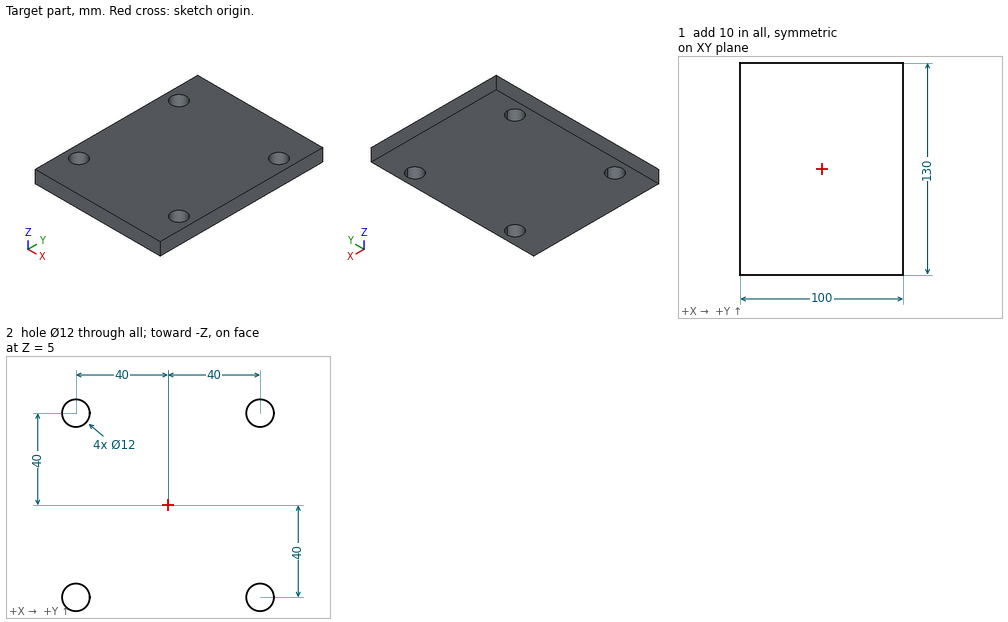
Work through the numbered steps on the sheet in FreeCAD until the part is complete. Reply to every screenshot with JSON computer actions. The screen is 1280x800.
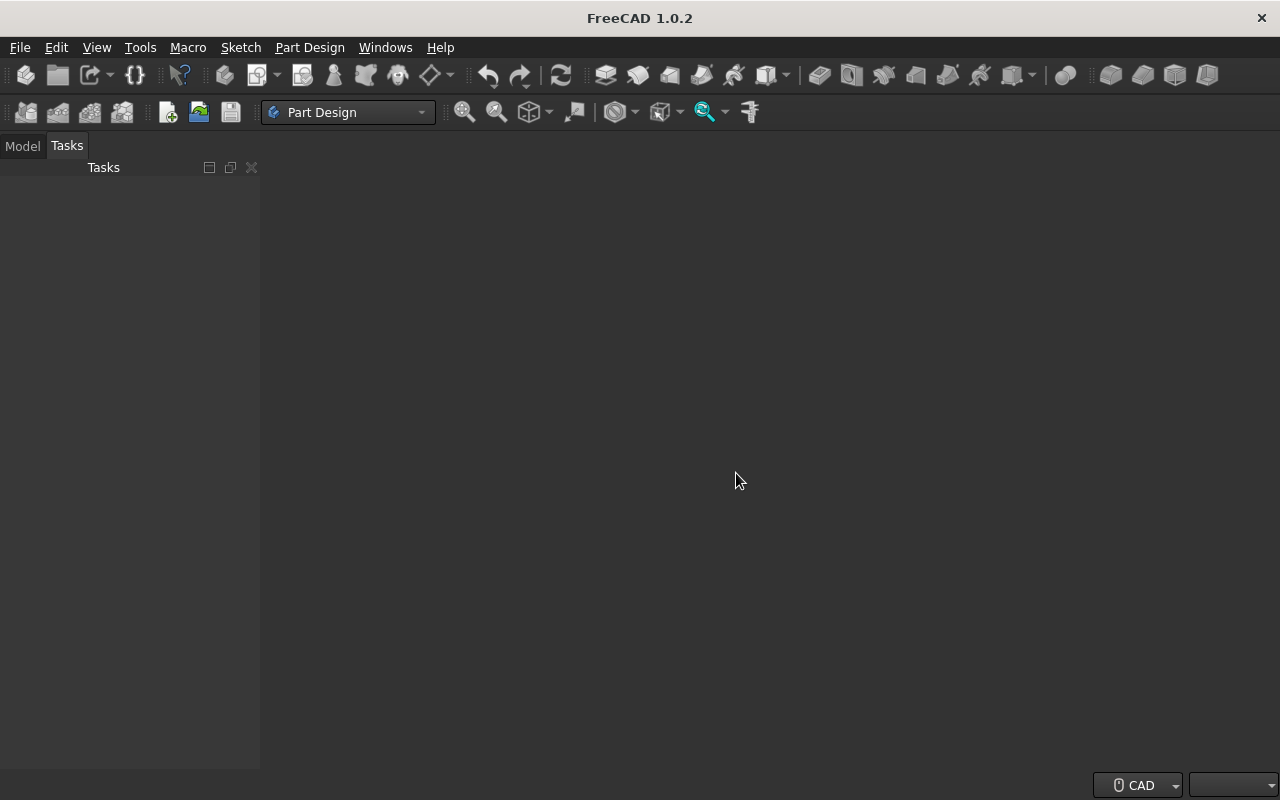
{"action": "left_click", "coordinate": [168, 112]}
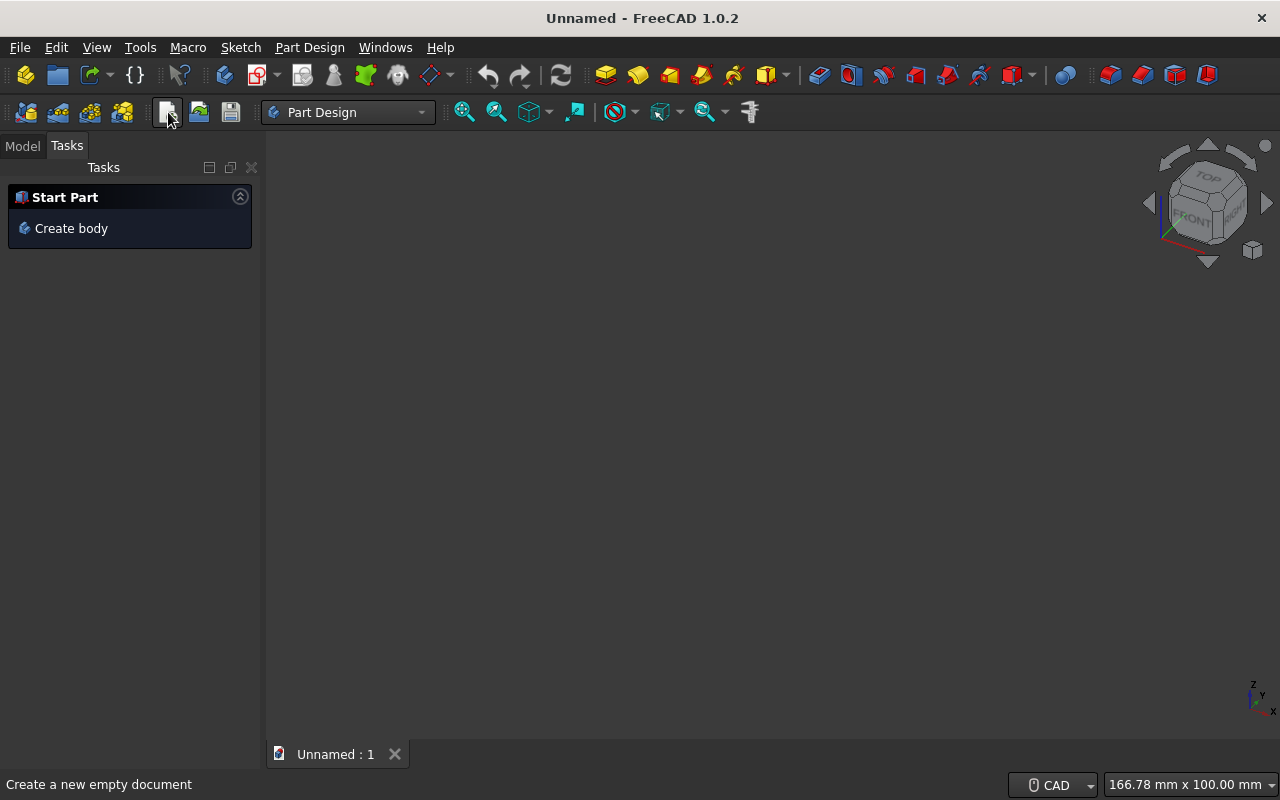
{"action": "left_click", "coordinate": [258, 76]}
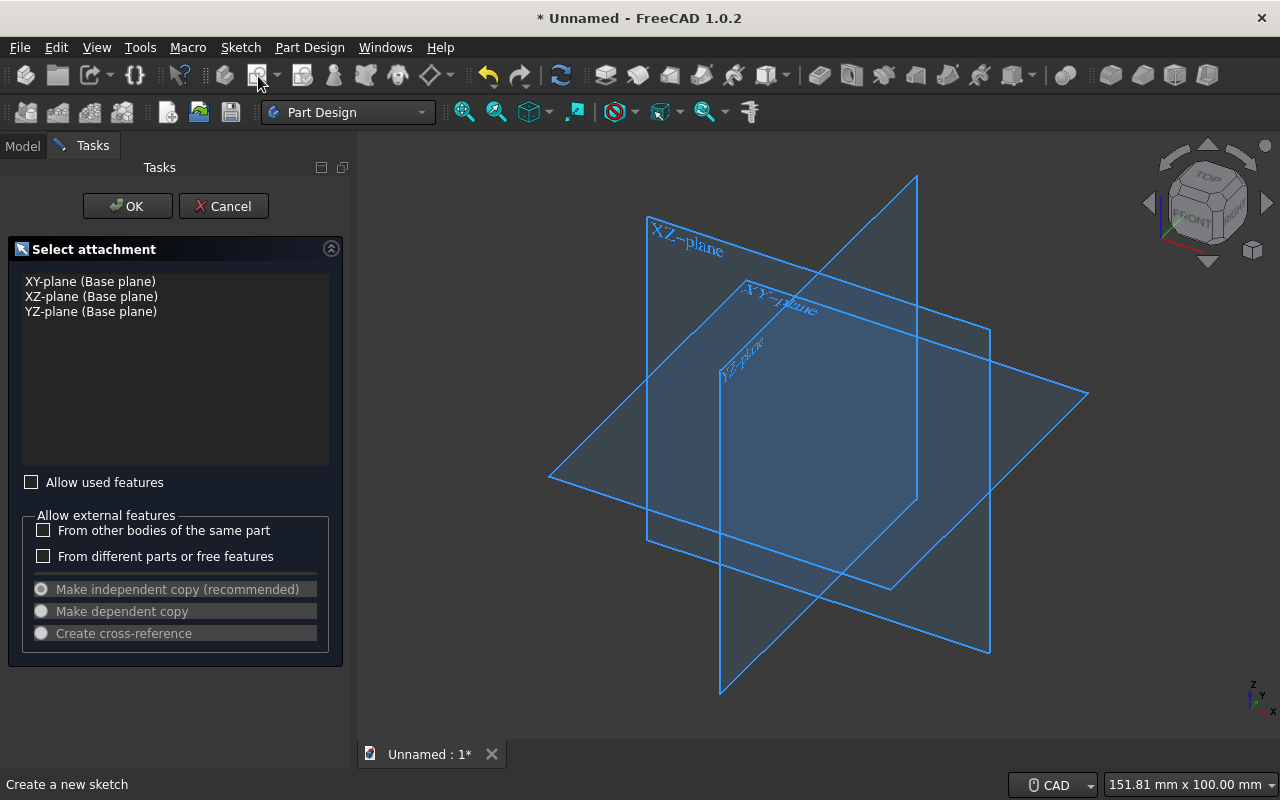
{"action": "left_click", "coordinate": [82, 282]}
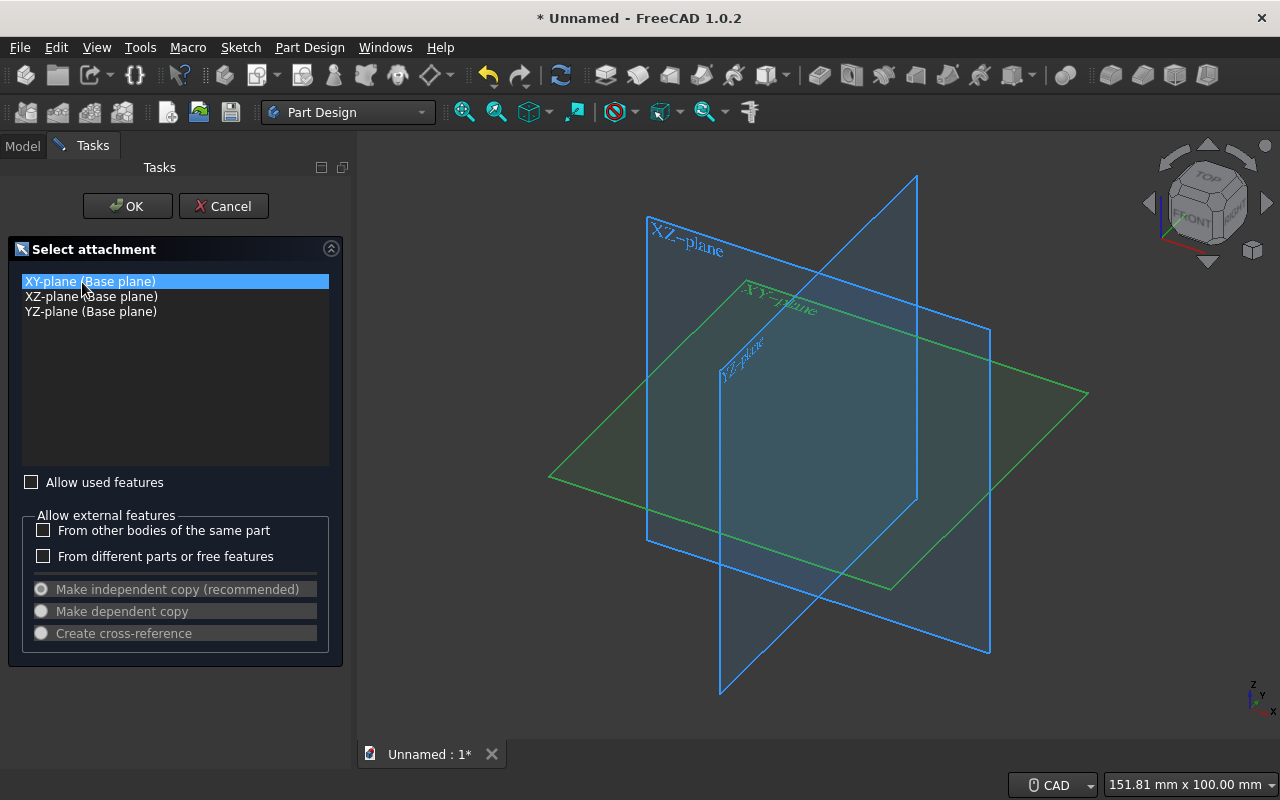
{"action": "left_click", "coordinate": [128, 206]}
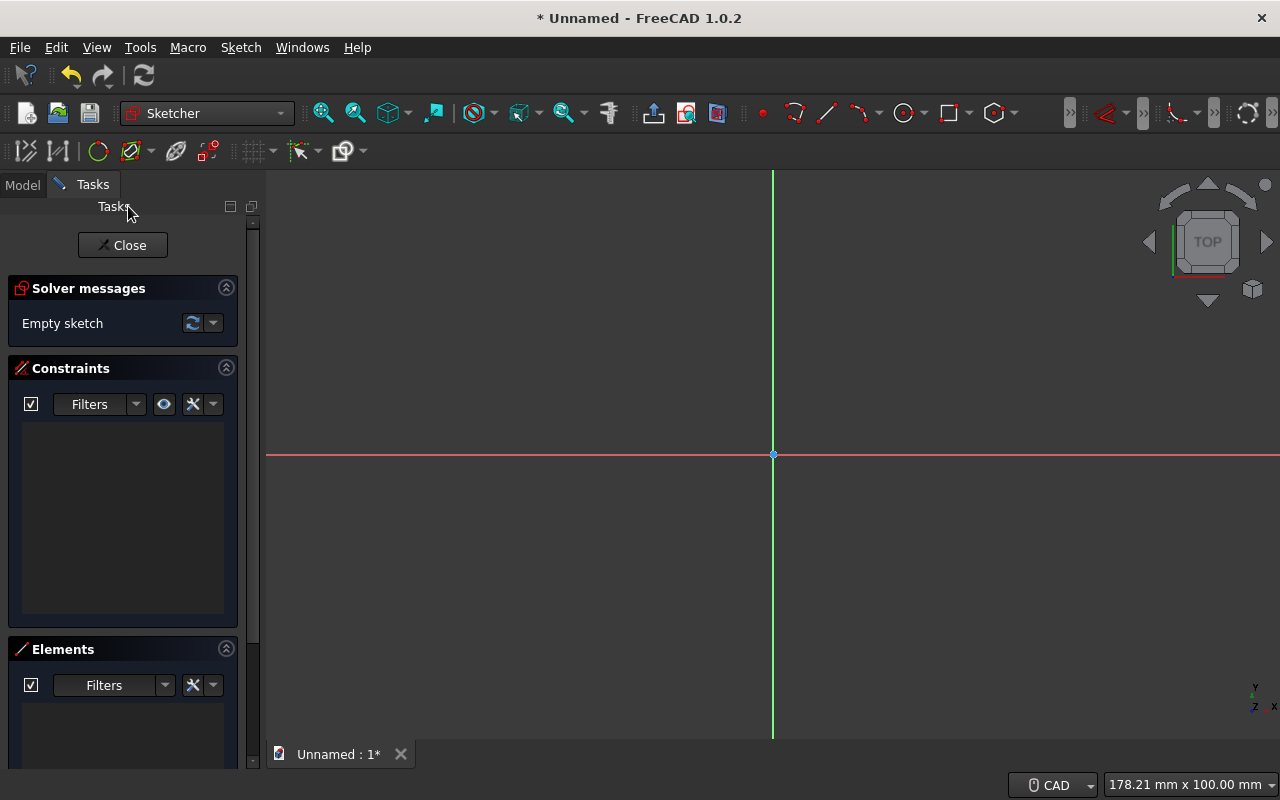
{"action": "scroll", "coordinate": [649, 454], "scroll_direction": "down", "scroll_amount": 4}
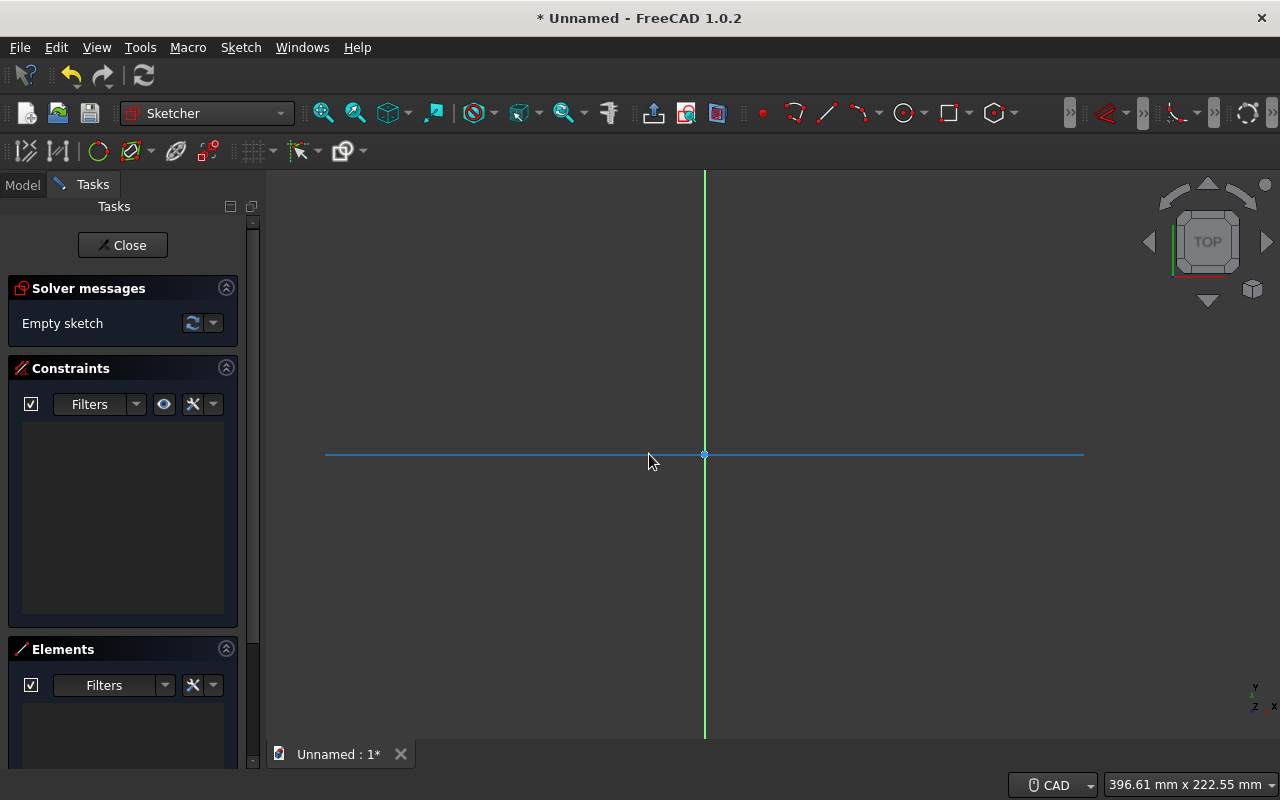
{"action": "key", "text": "g v"}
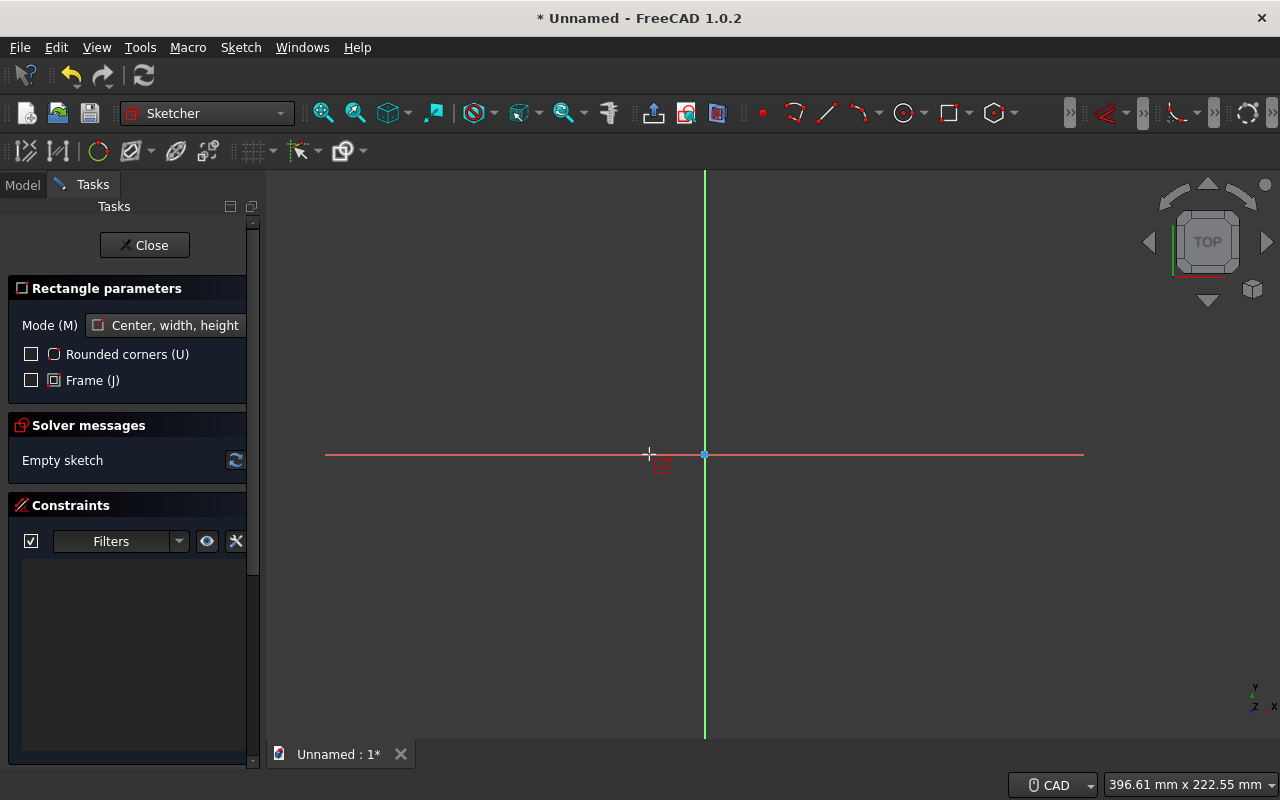
{"action": "left_click", "coordinate": [705, 454]}
{"action": "left_click", "coordinate": [833, 288]}
{"action": "key", "text": "Escape"}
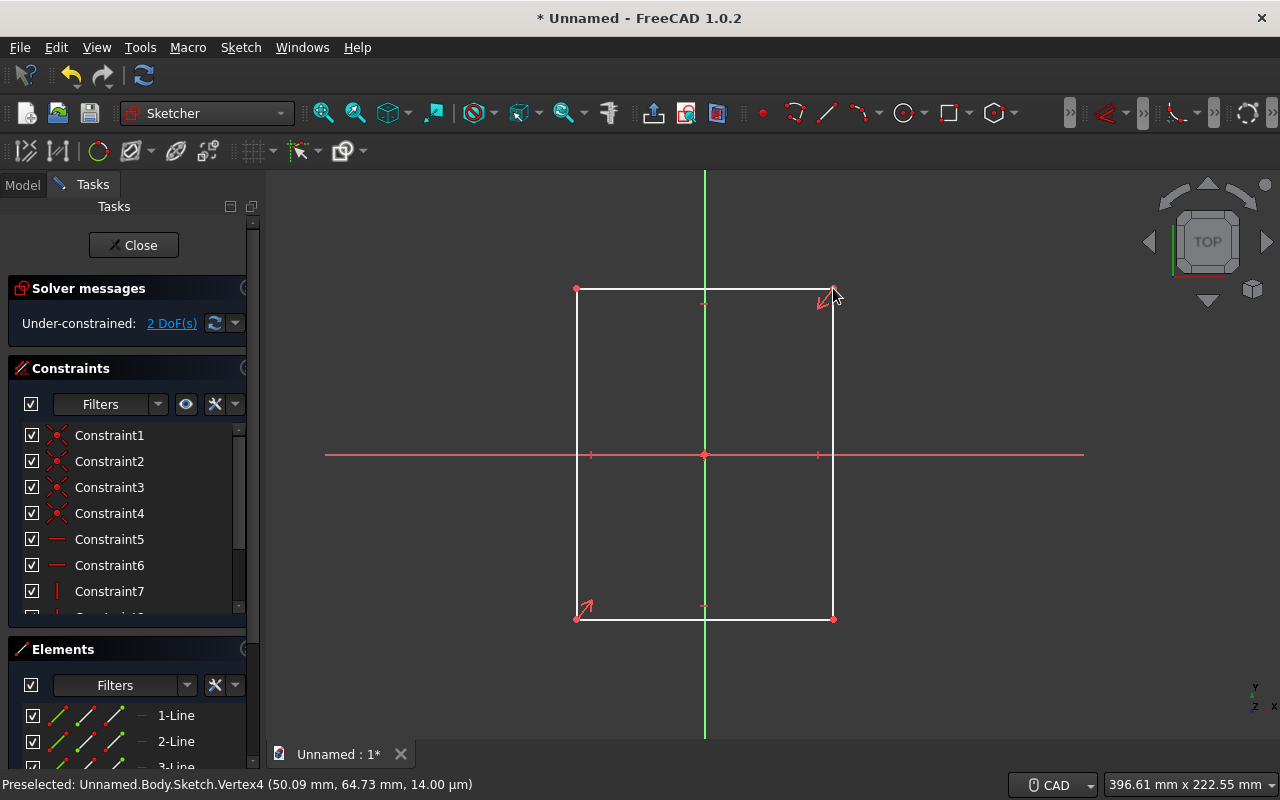
{"action": "left_click", "coordinate": [654, 620]}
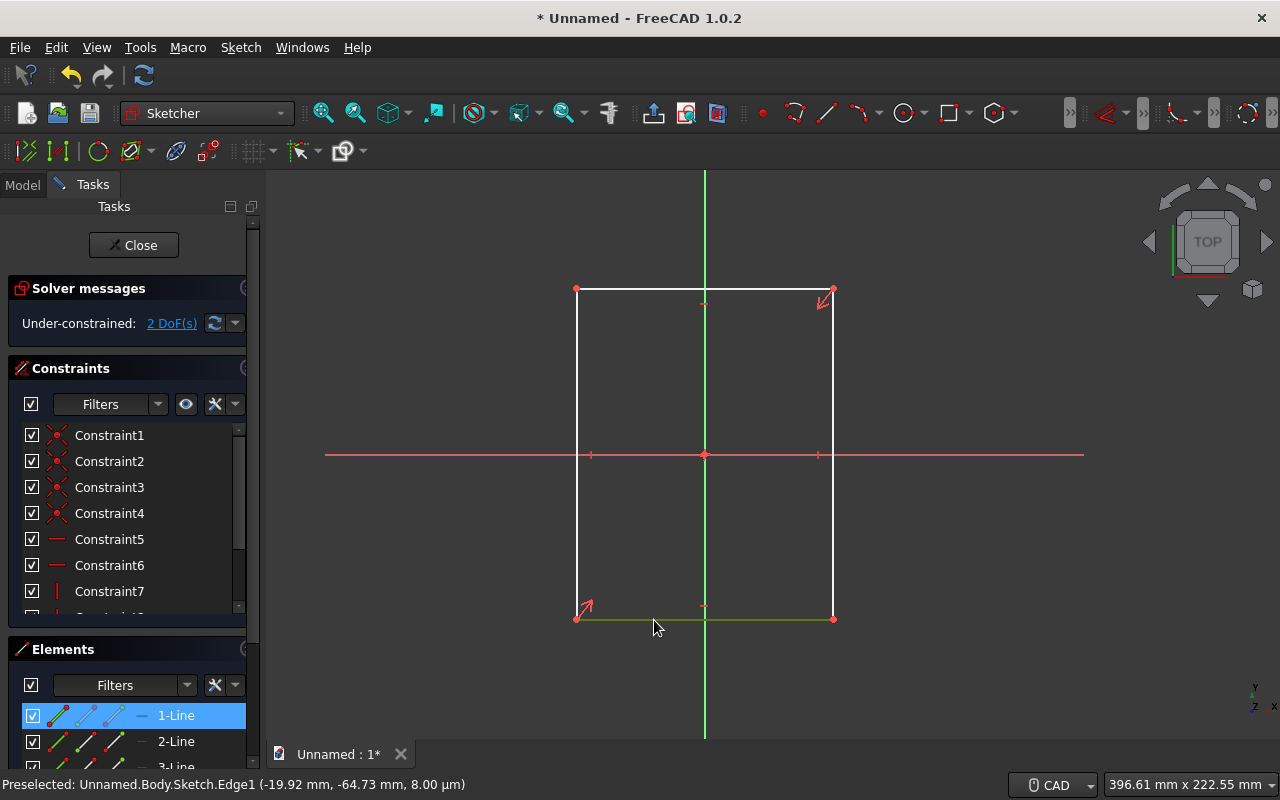
{"action": "left_click", "coordinate": [1128, 114]}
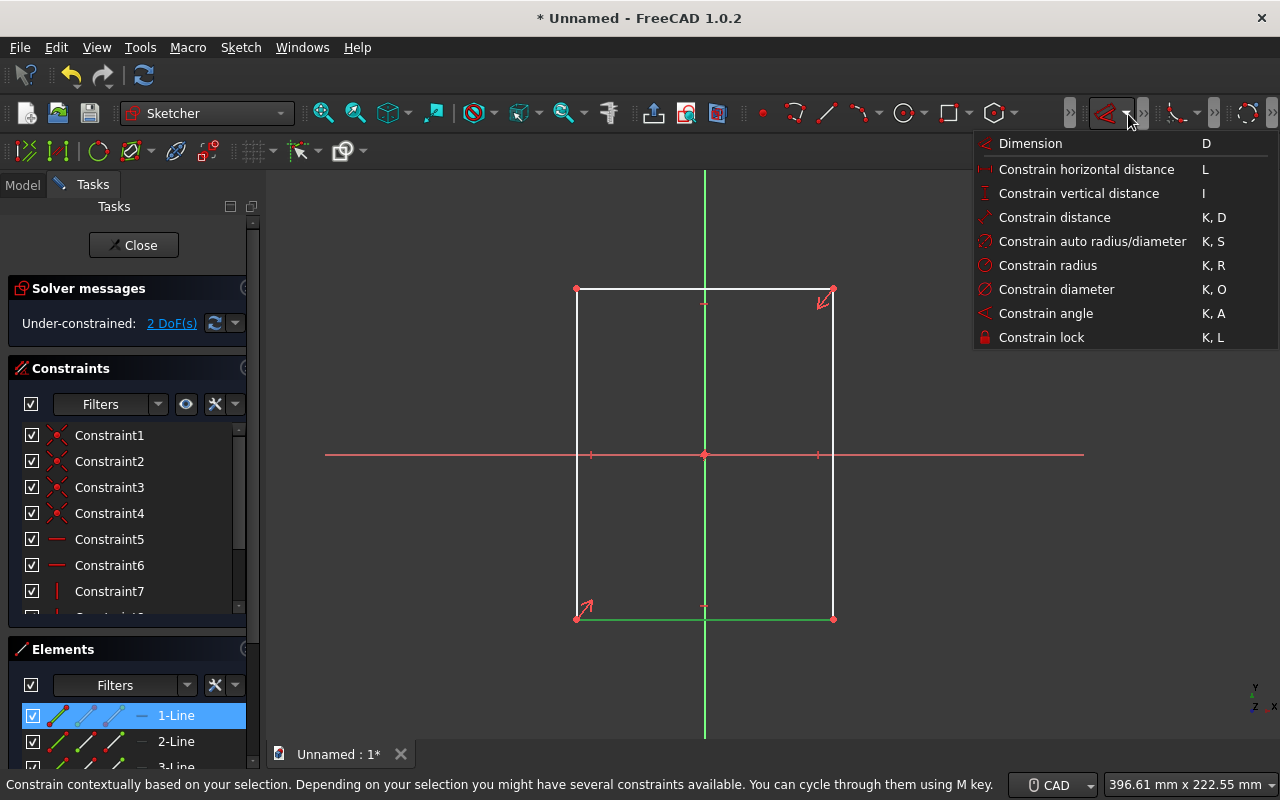
{"action": "left_click", "coordinate": [1126, 169]}